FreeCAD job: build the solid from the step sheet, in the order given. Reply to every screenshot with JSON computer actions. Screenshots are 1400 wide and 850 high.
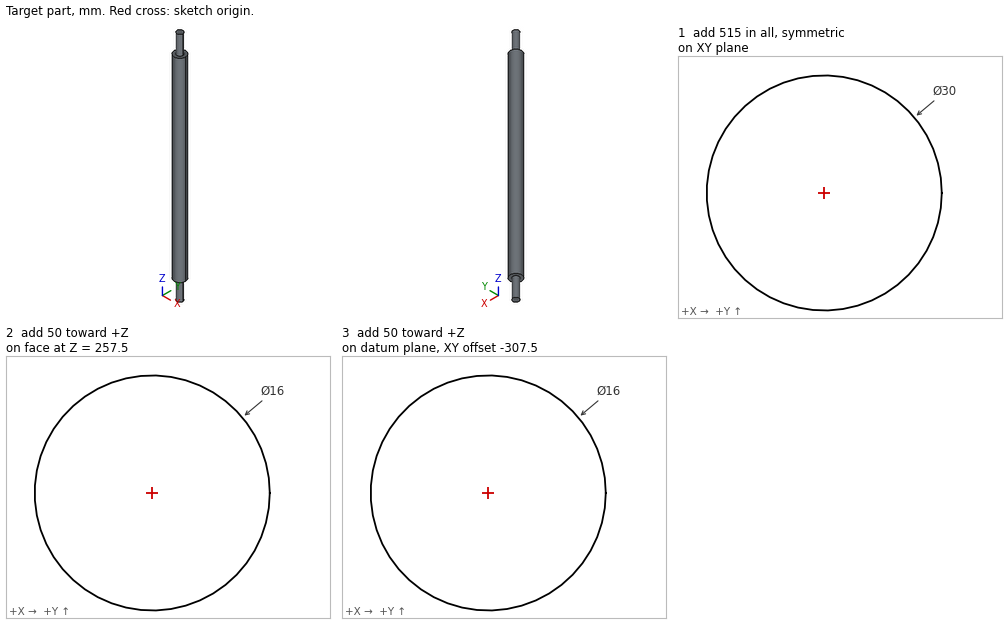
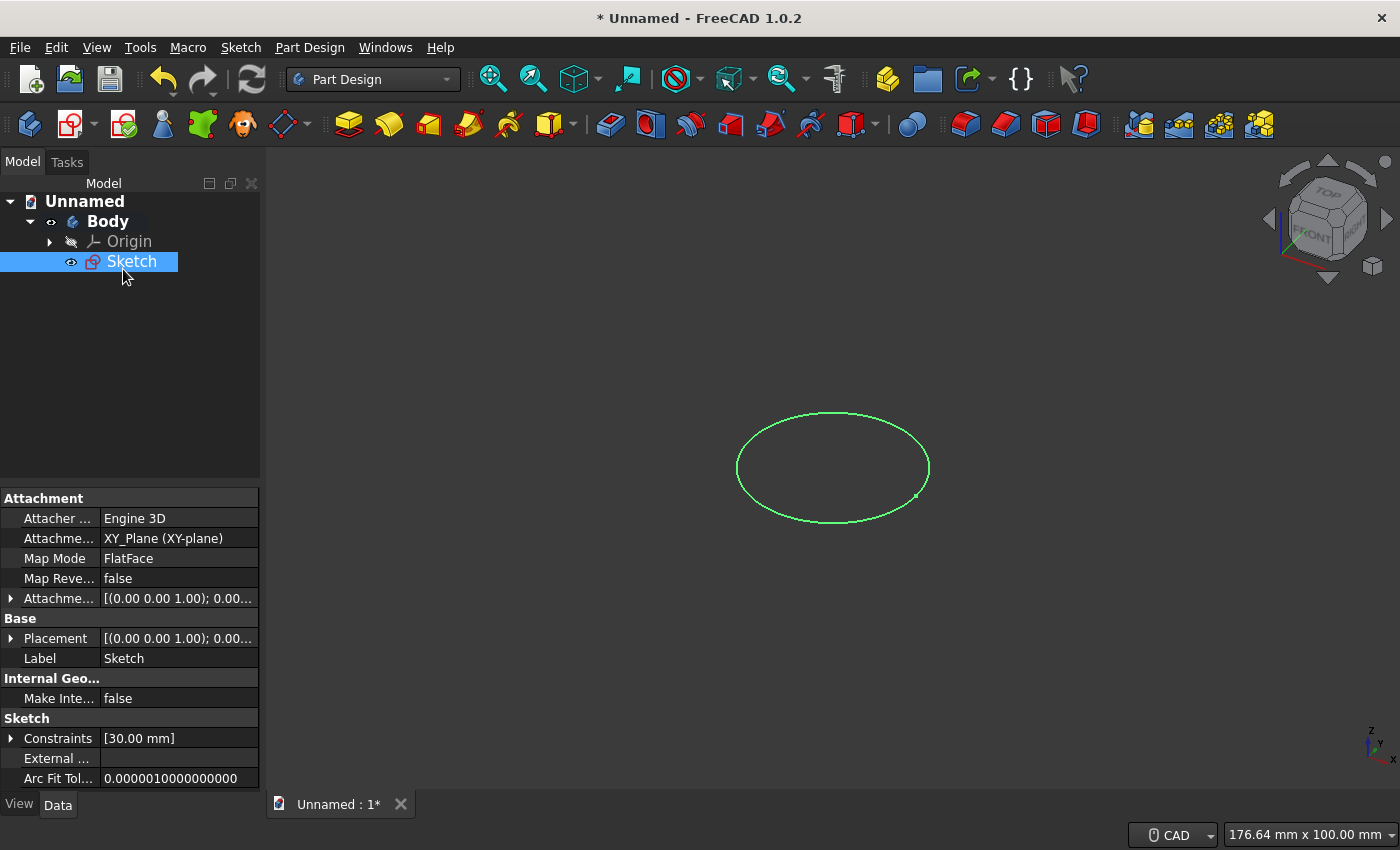
{"action": "left_click", "coordinate": [350, 124]}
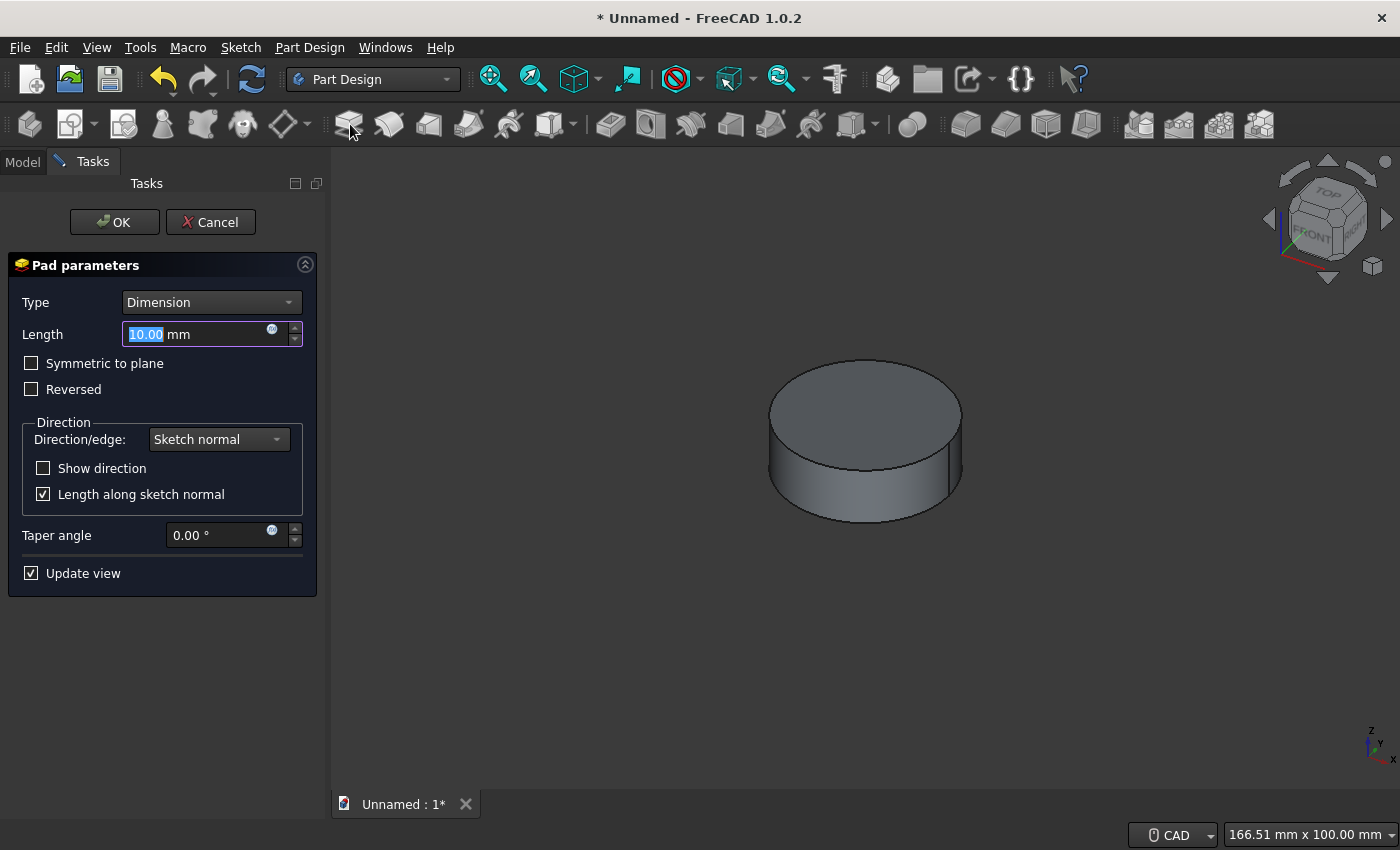
{"action": "type", "text": "515"}
{"action": "key", "text": "Tab"}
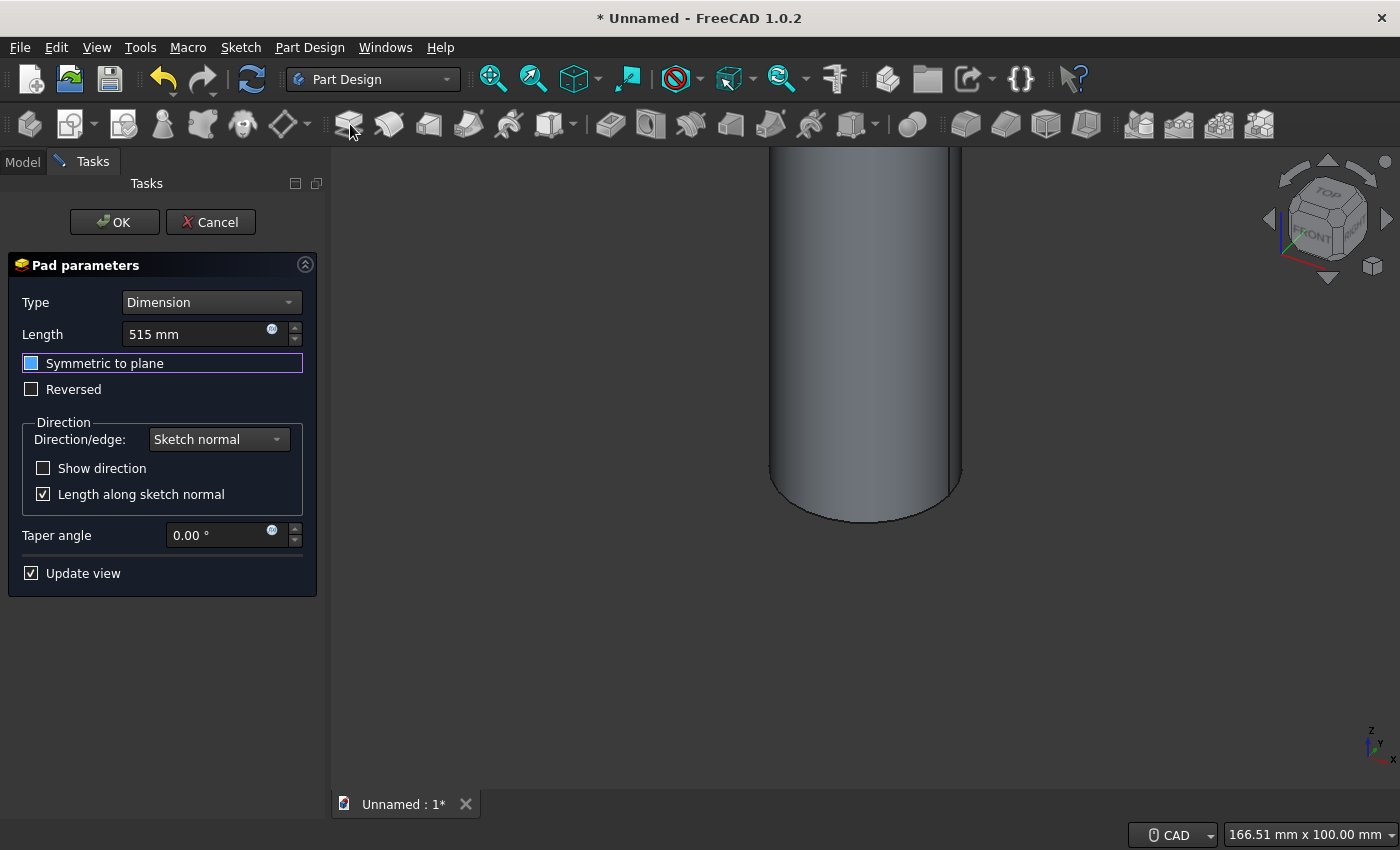
{"action": "left_click", "coordinate": [30, 363]}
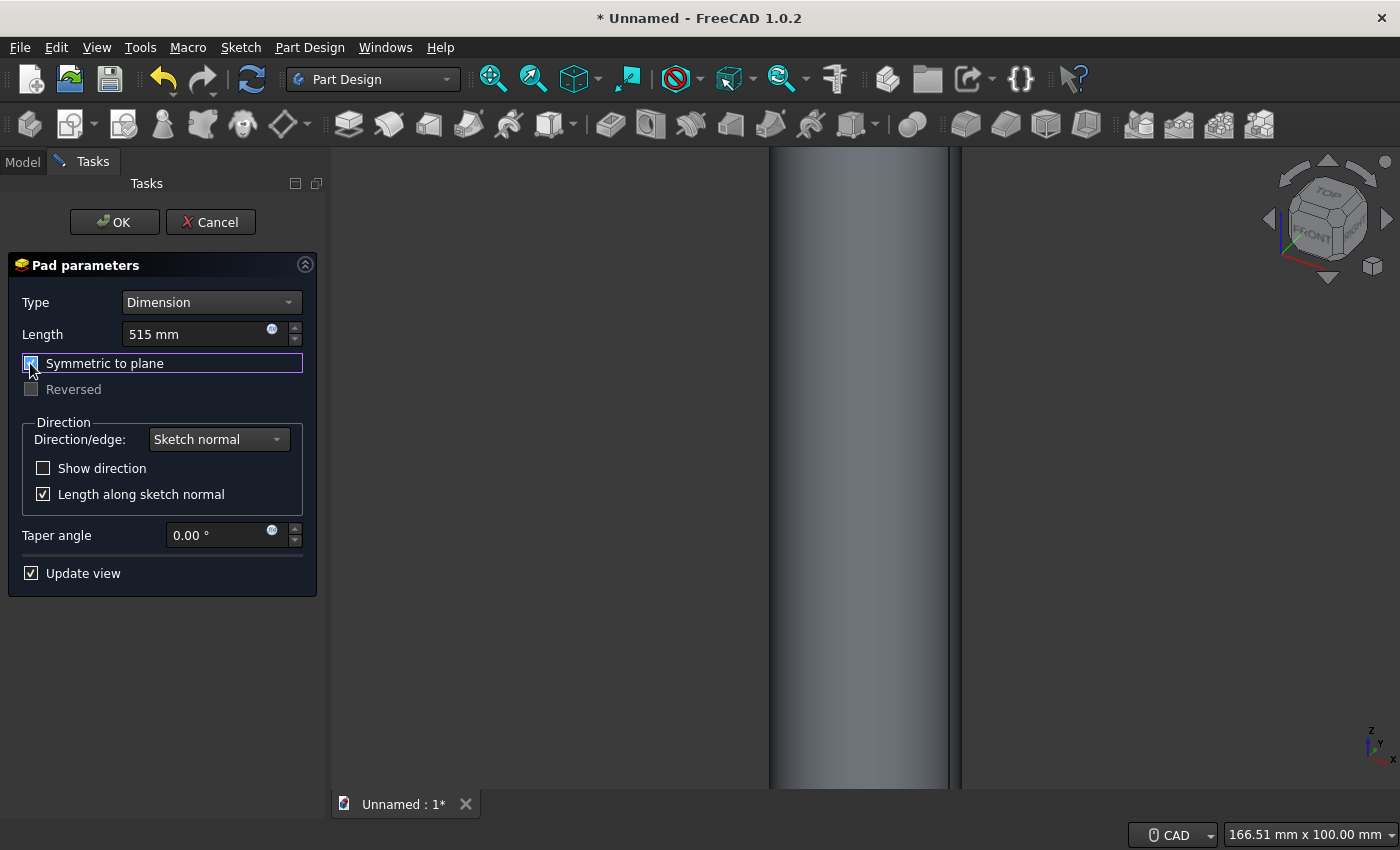
{"action": "left_click", "coordinate": [115, 222]}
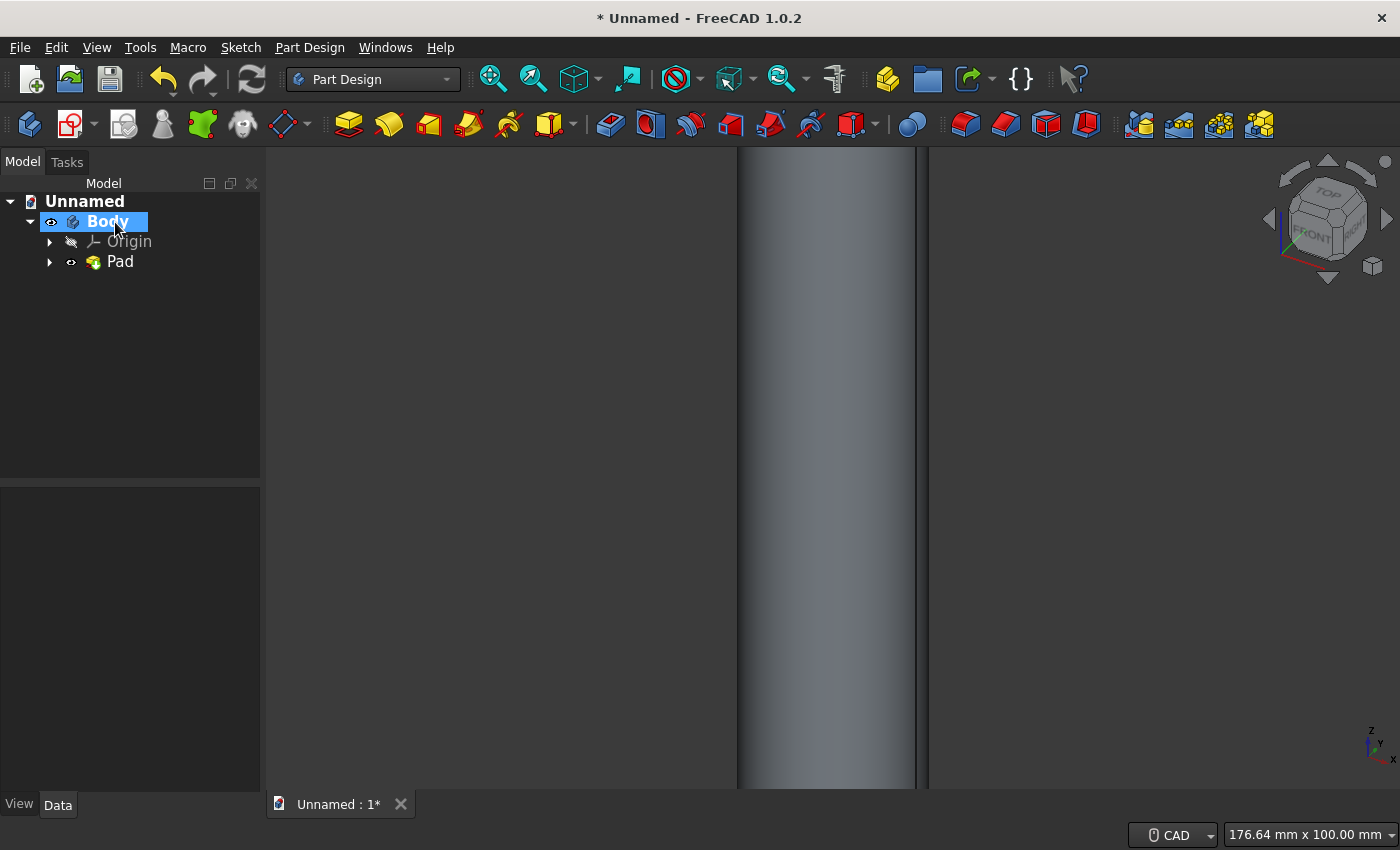
{"action": "key", "text": "v f"}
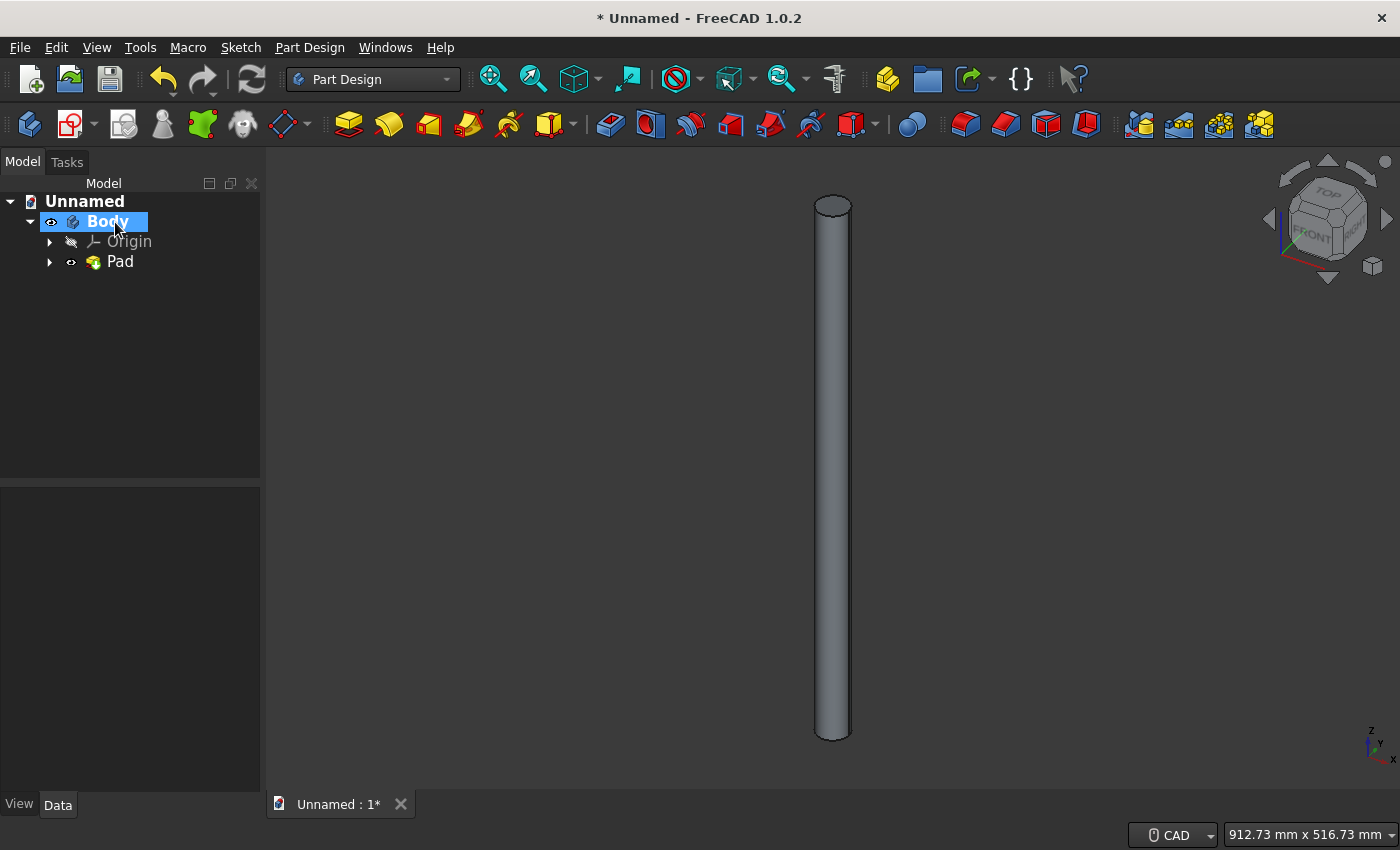
{"action": "left_click", "coordinate": [833, 205]}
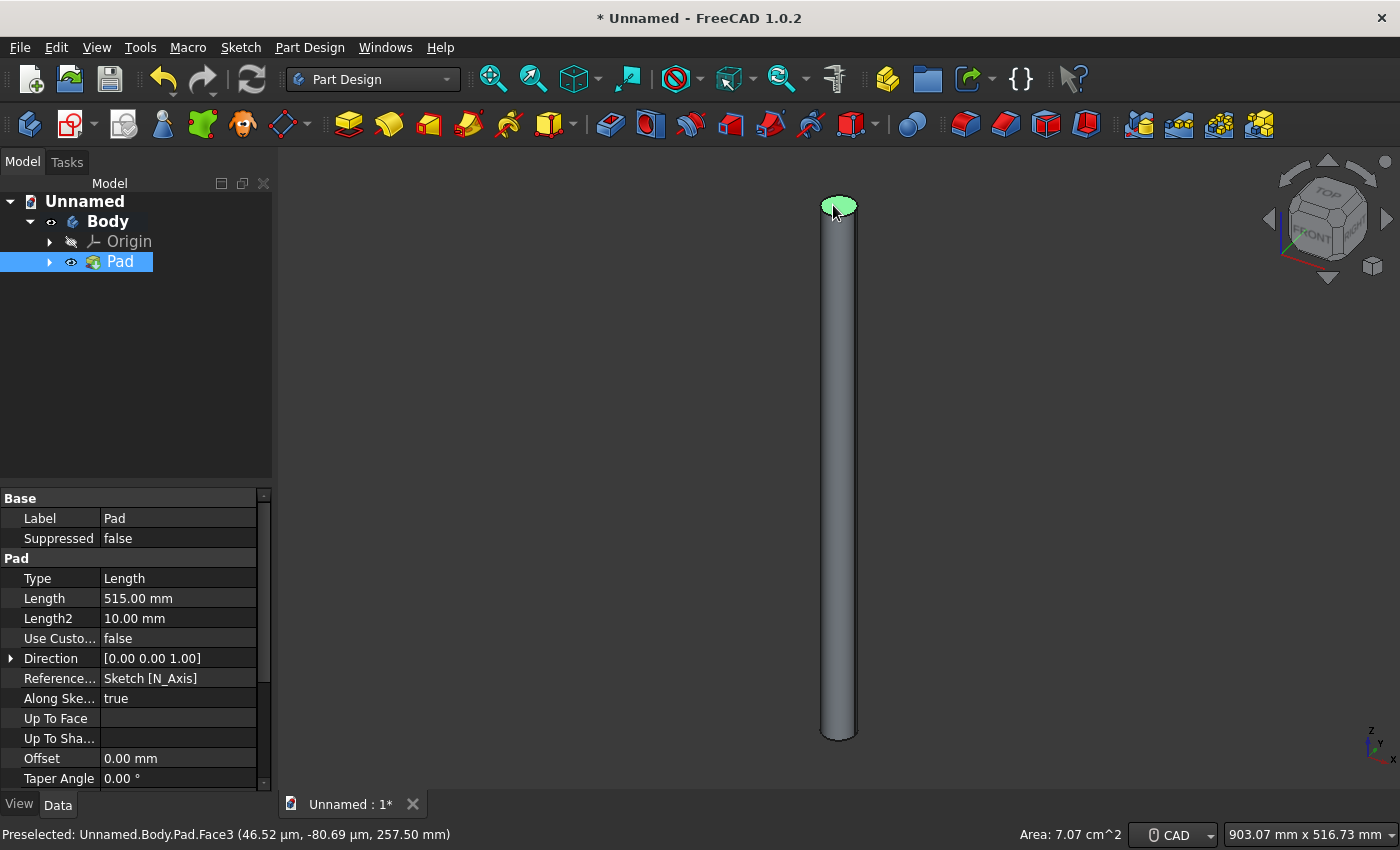
{"action": "left_click", "coordinate": [70, 124]}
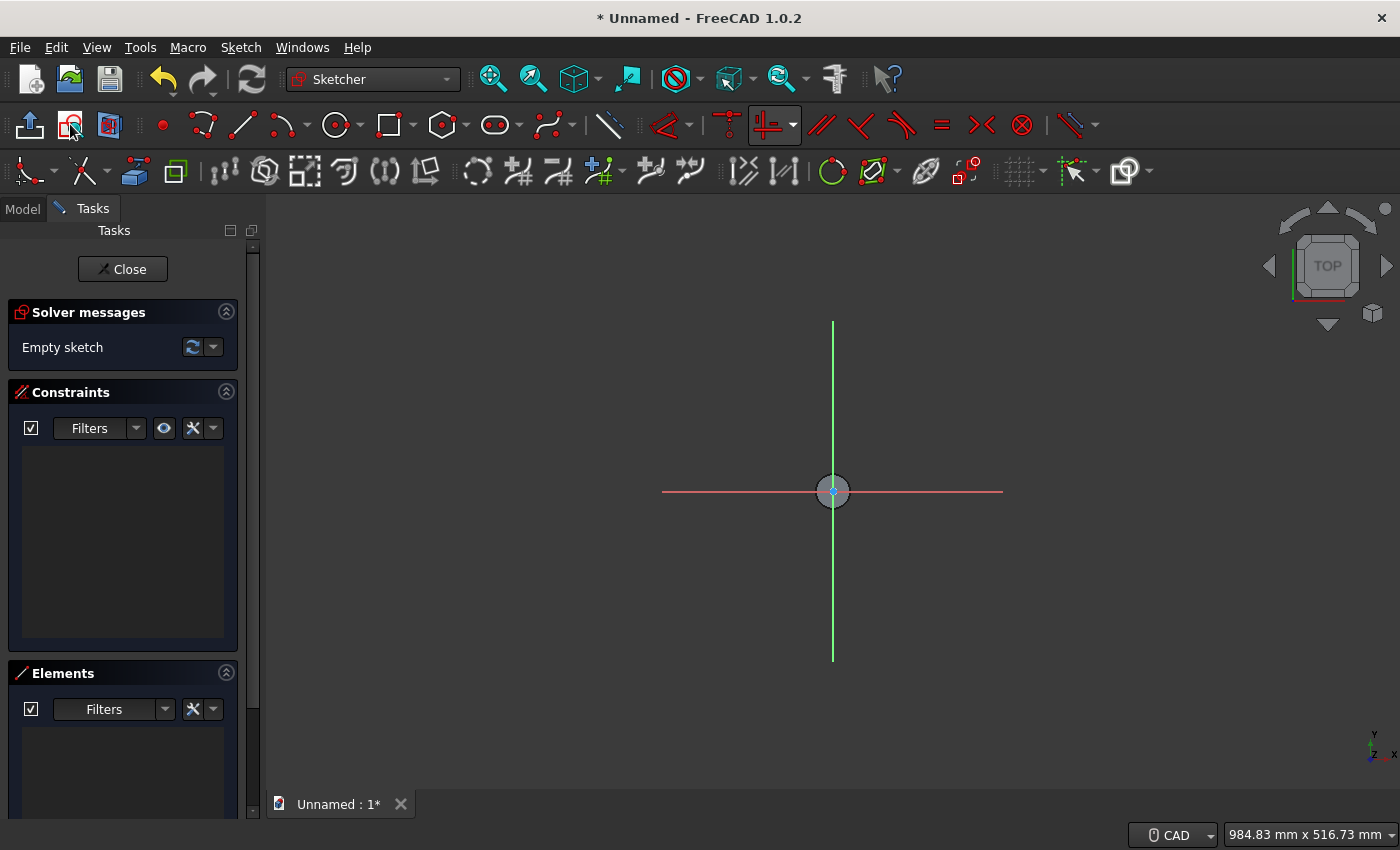
{"action": "scroll", "coordinate": [837, 492], "scroll_direction": "up", "scroll_amount": 15}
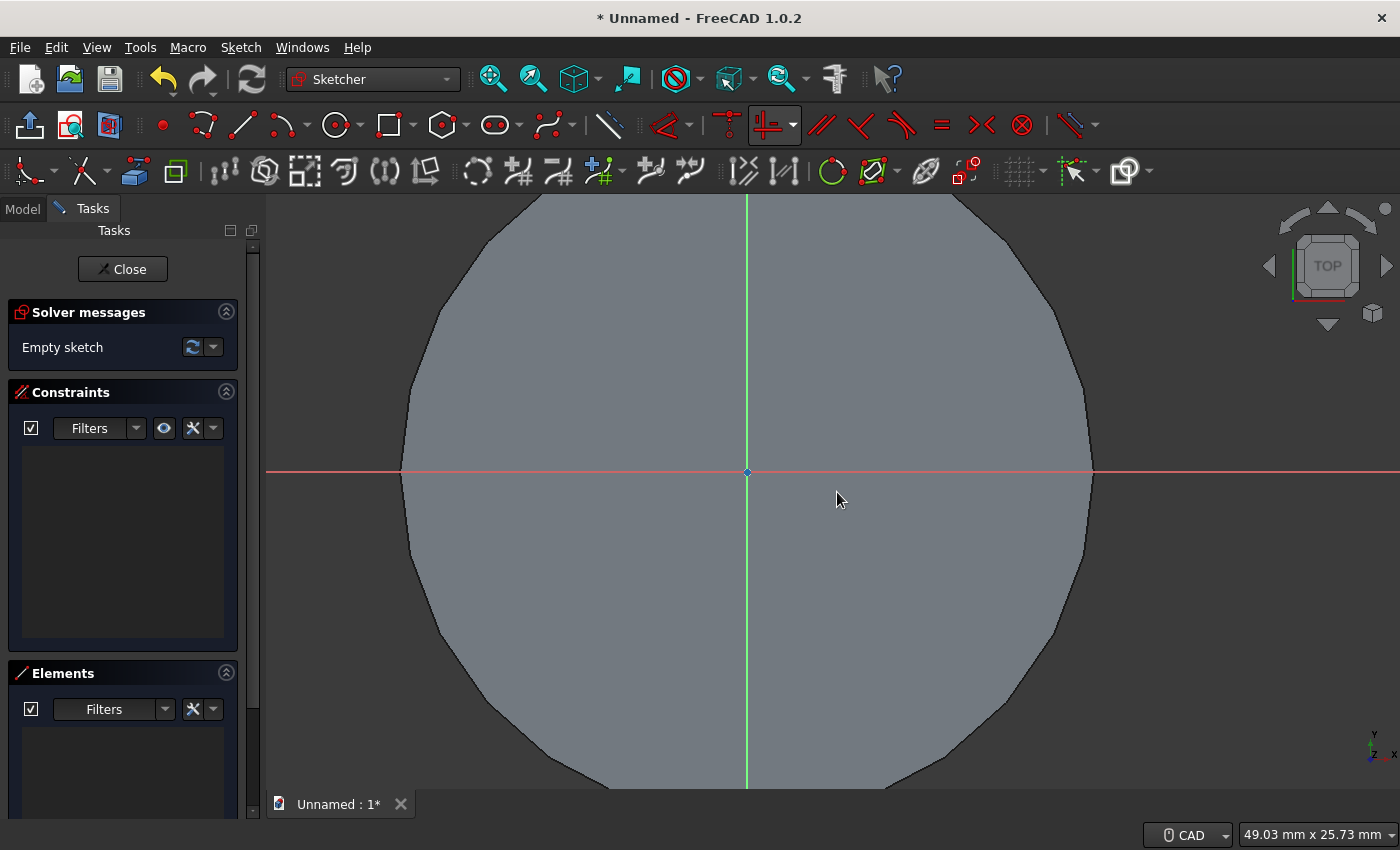
{"action": "left_click", "coordinate": [336, 126]}